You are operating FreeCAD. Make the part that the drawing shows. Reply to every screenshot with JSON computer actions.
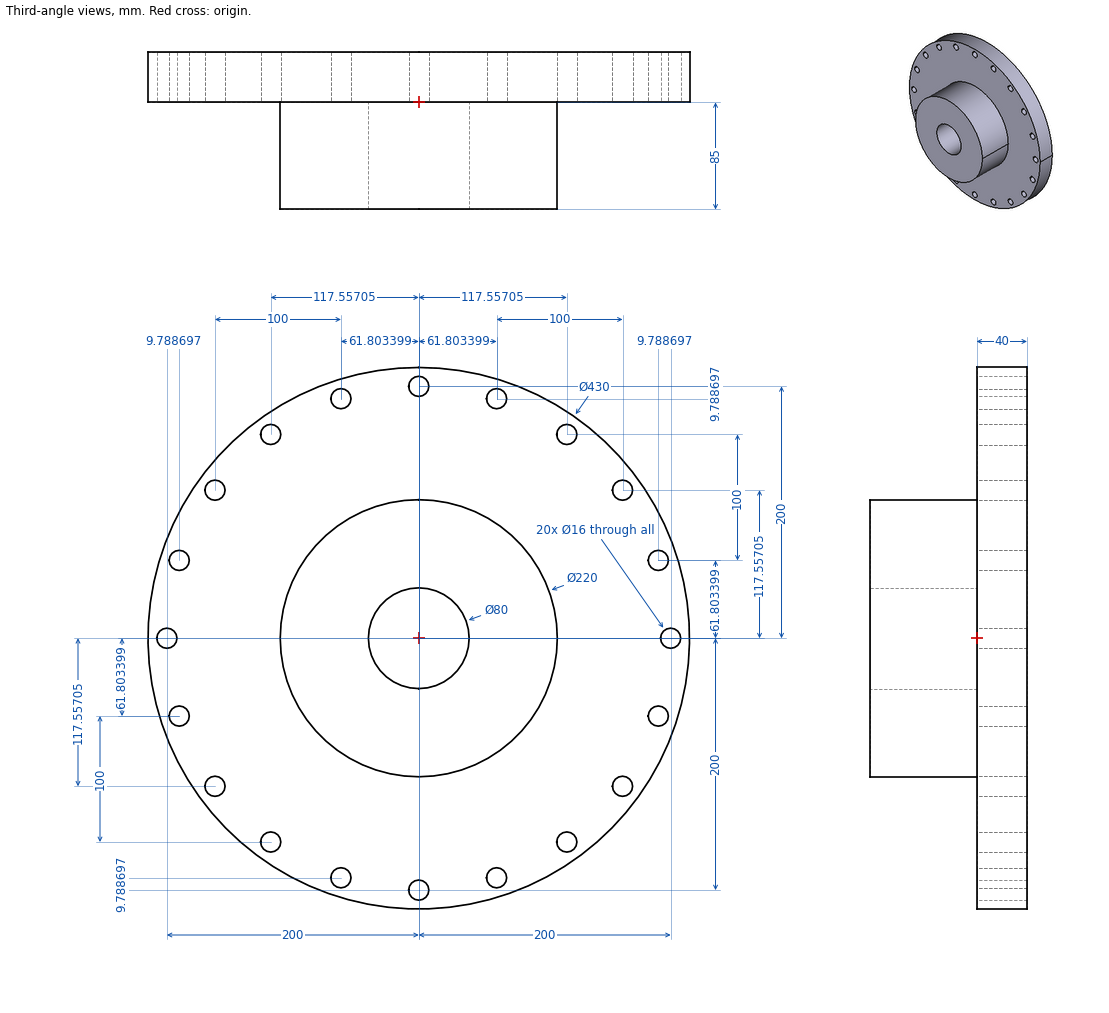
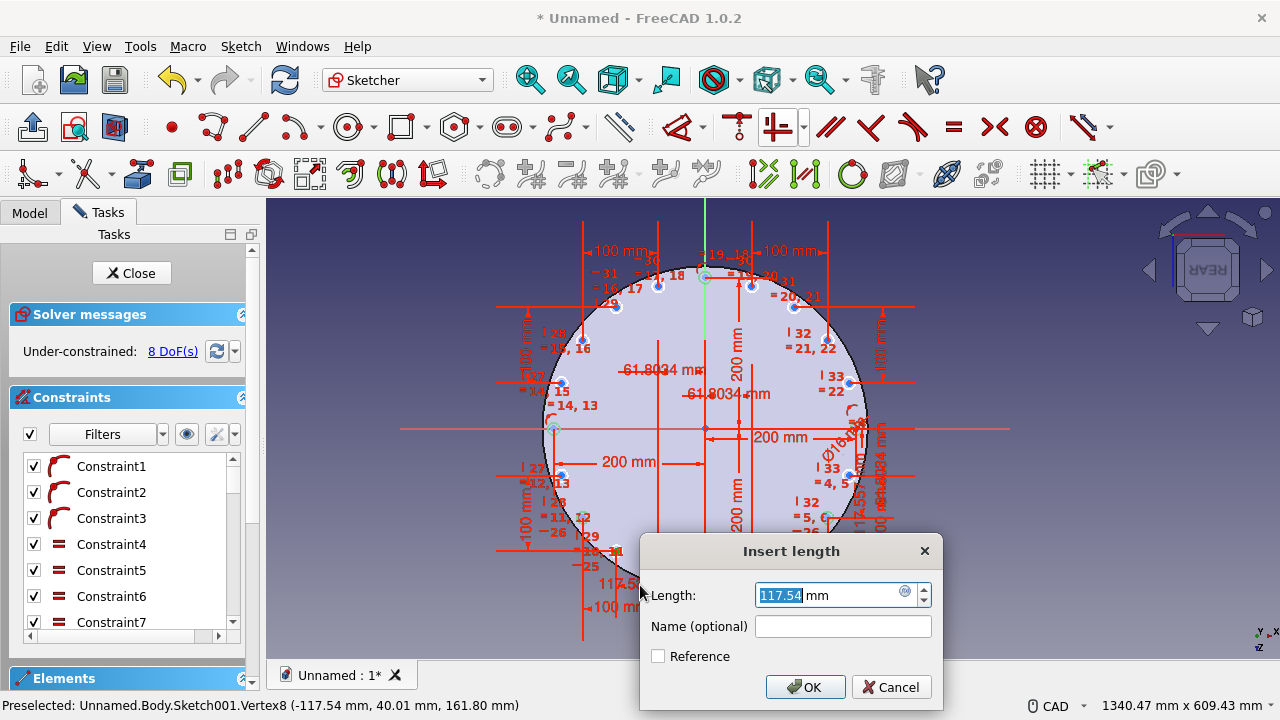
{"action": "type", "text": "117.55705"}
{"action": "key", "text": "Return"}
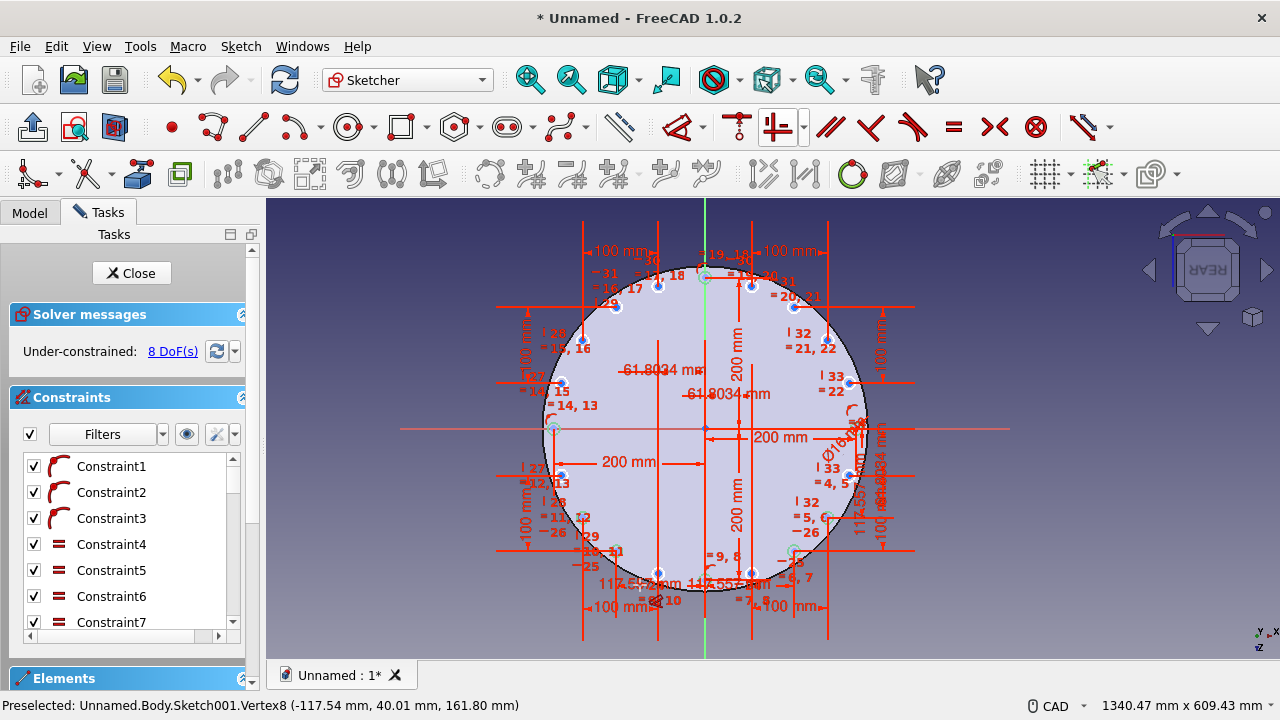
{"action": "left_click", "coordinate": [562, 383]}
{"action": "left_click", "coordinate": [528, 406]}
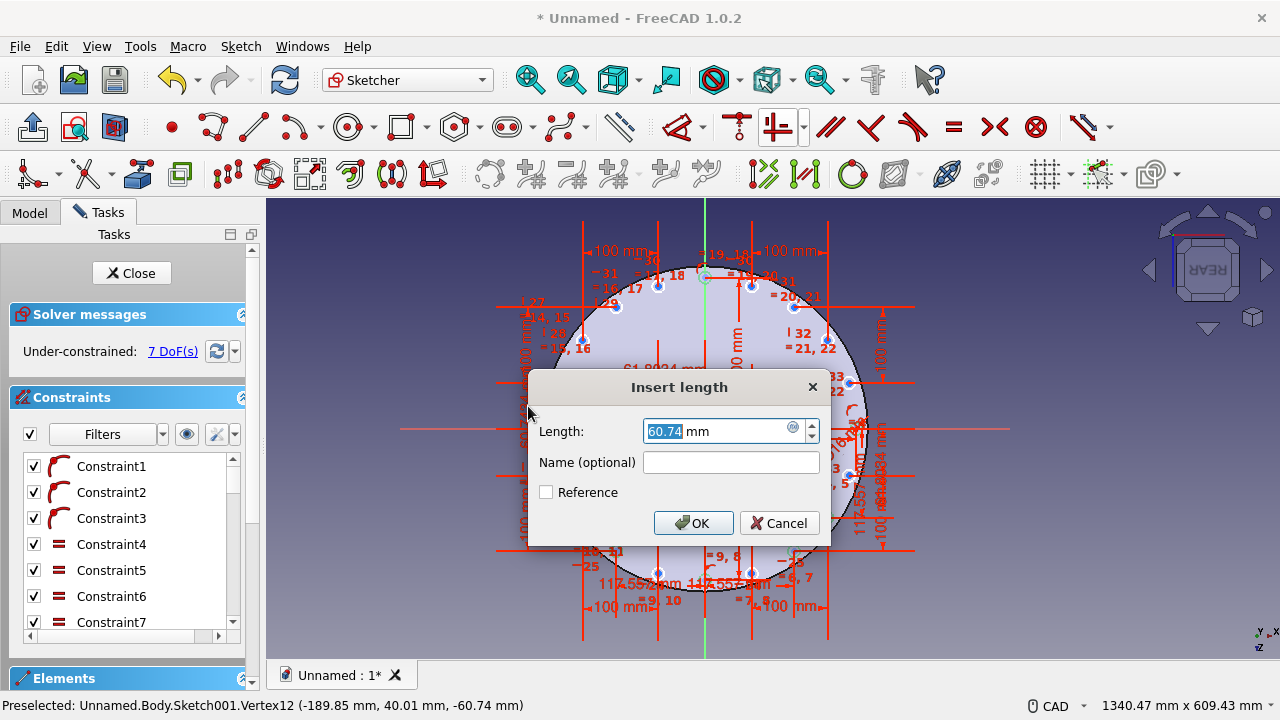
{"action": "type", "text": "61.803399"}
{"action": "key", "text": "Return"}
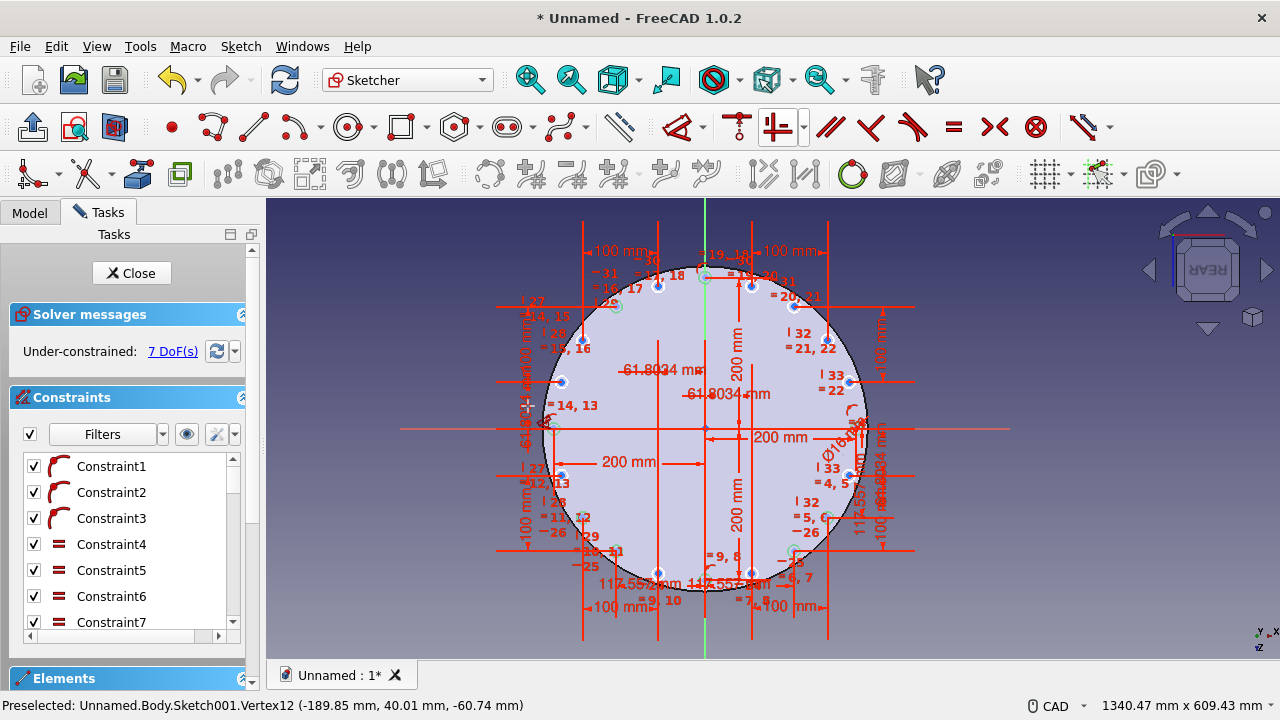
{"action": "left_click", "coordinate": [583, 341]}
{"action": "left_click", "coordinate": [739, 416]}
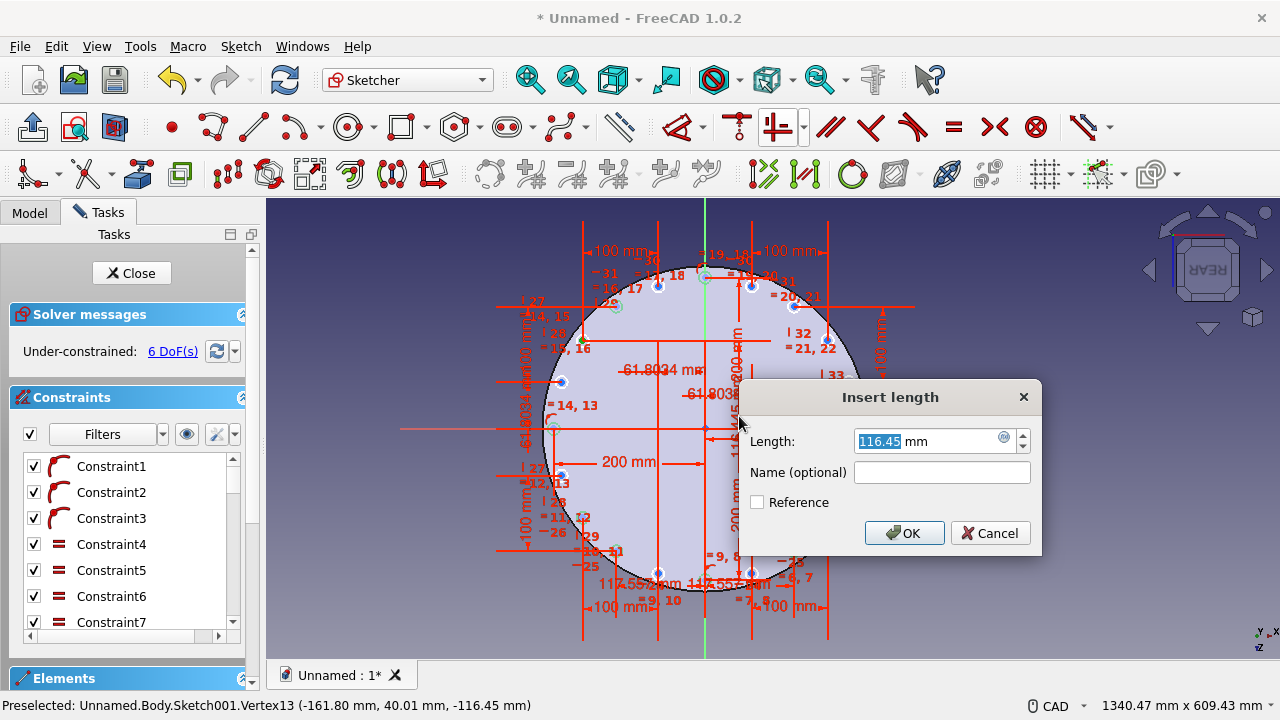
{"action": "type", "text": "117.55705"}
{"action": "key", "text": "Return"}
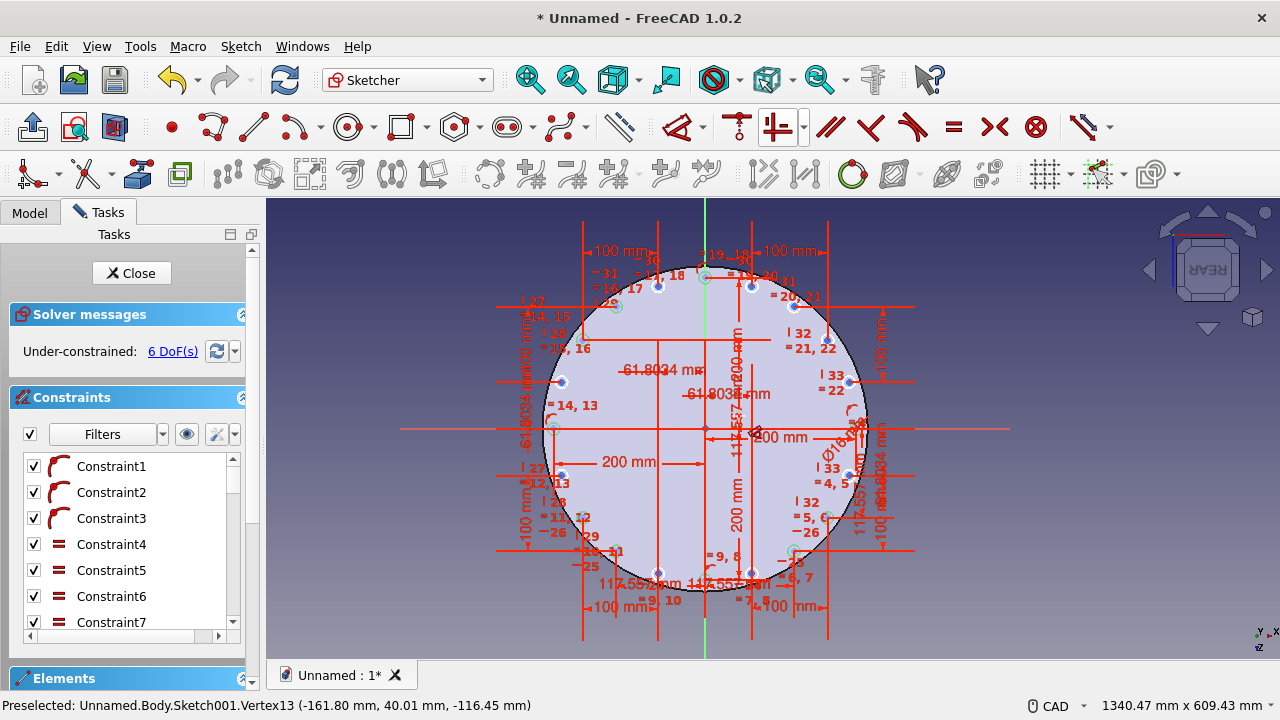
{"action": "left_click", "coordinate": [794, 307]}
{"action": "left_click", "coordinate": [729, 273]}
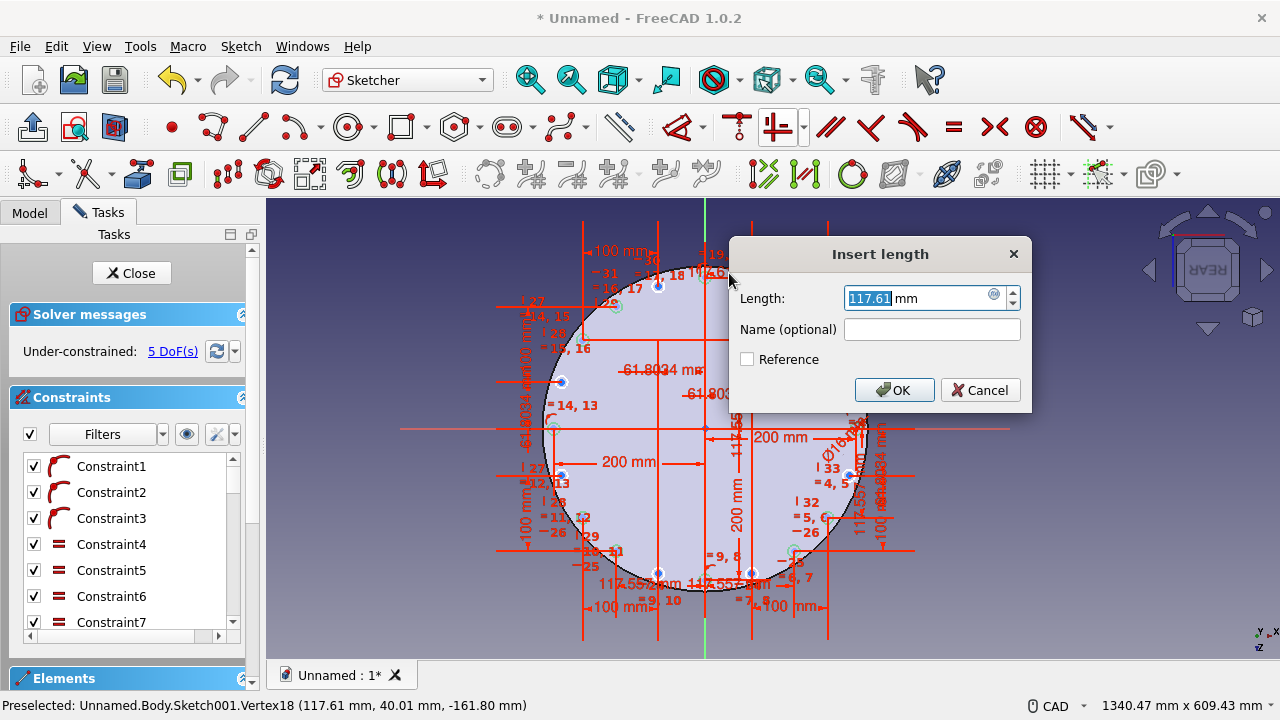
{"action": "type", "text": "117.55705"}
{"action": "key", "text": "Return"}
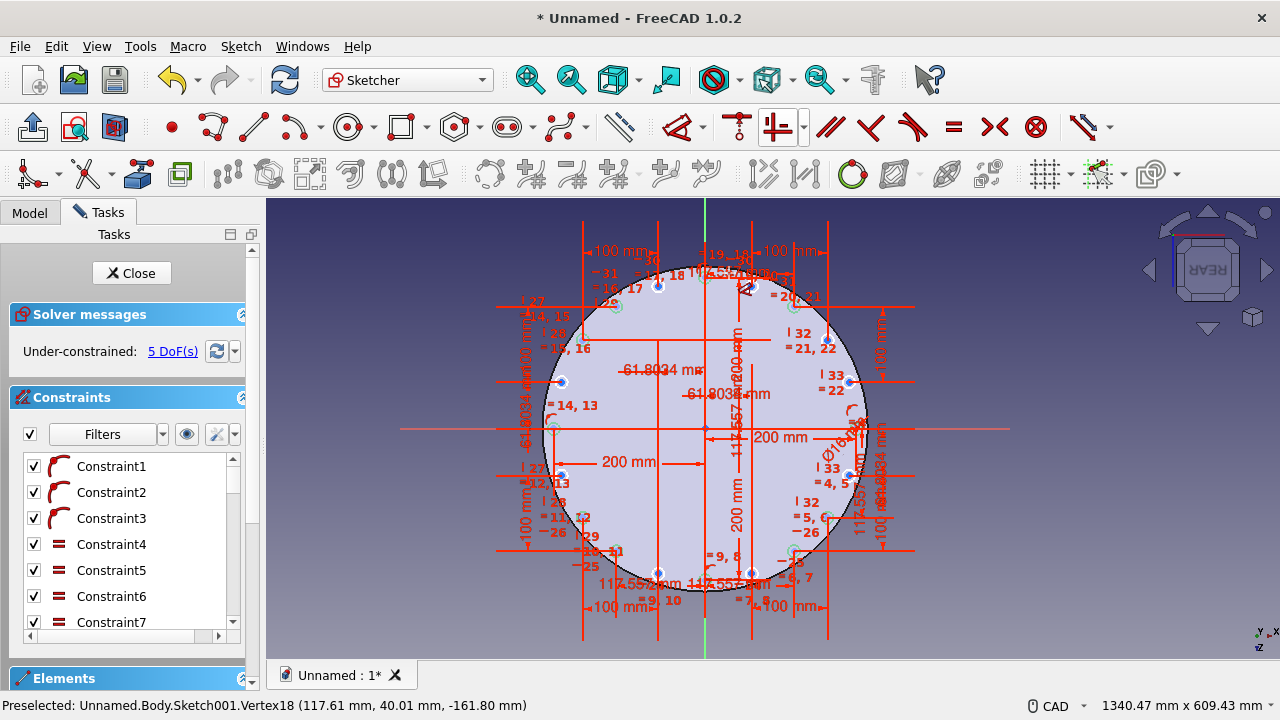
{"action": "left_click", "coordinate": [828, 340]}
{"action": "left_click", "coordinate": [862, 405]}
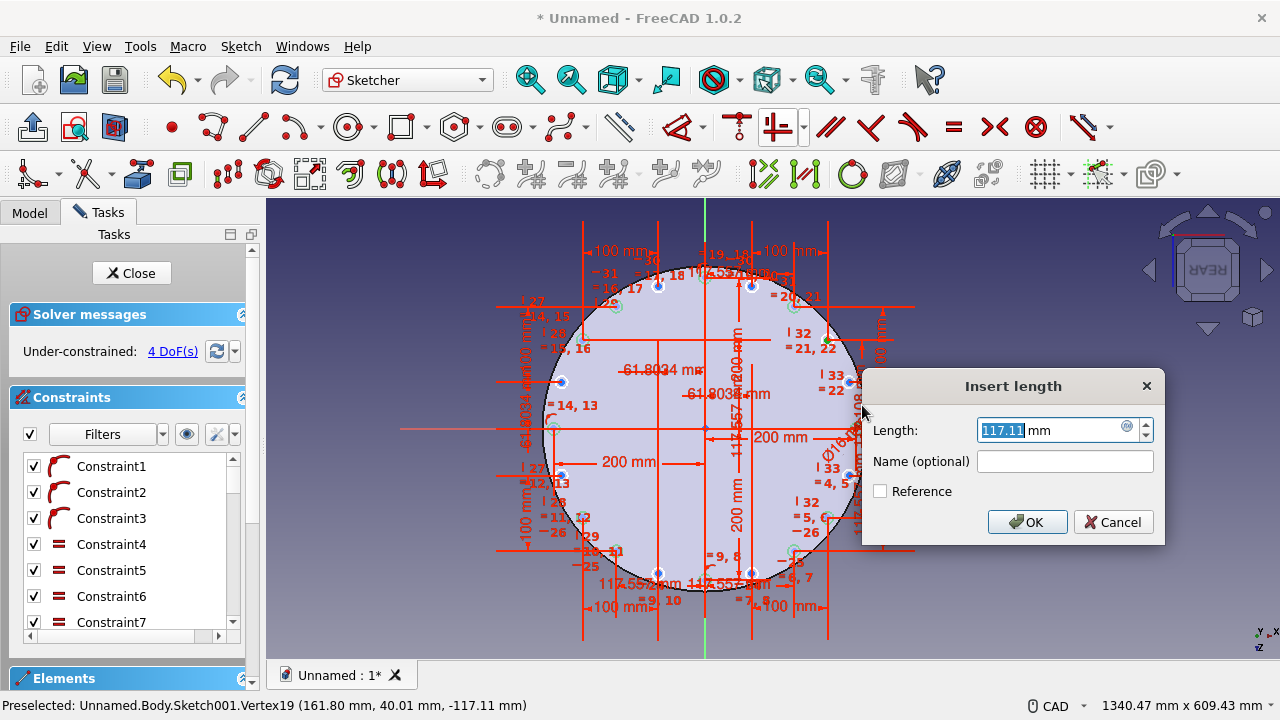
{"action": "type", "text": "117.55705"}
{"action": "key", "text": "Return"}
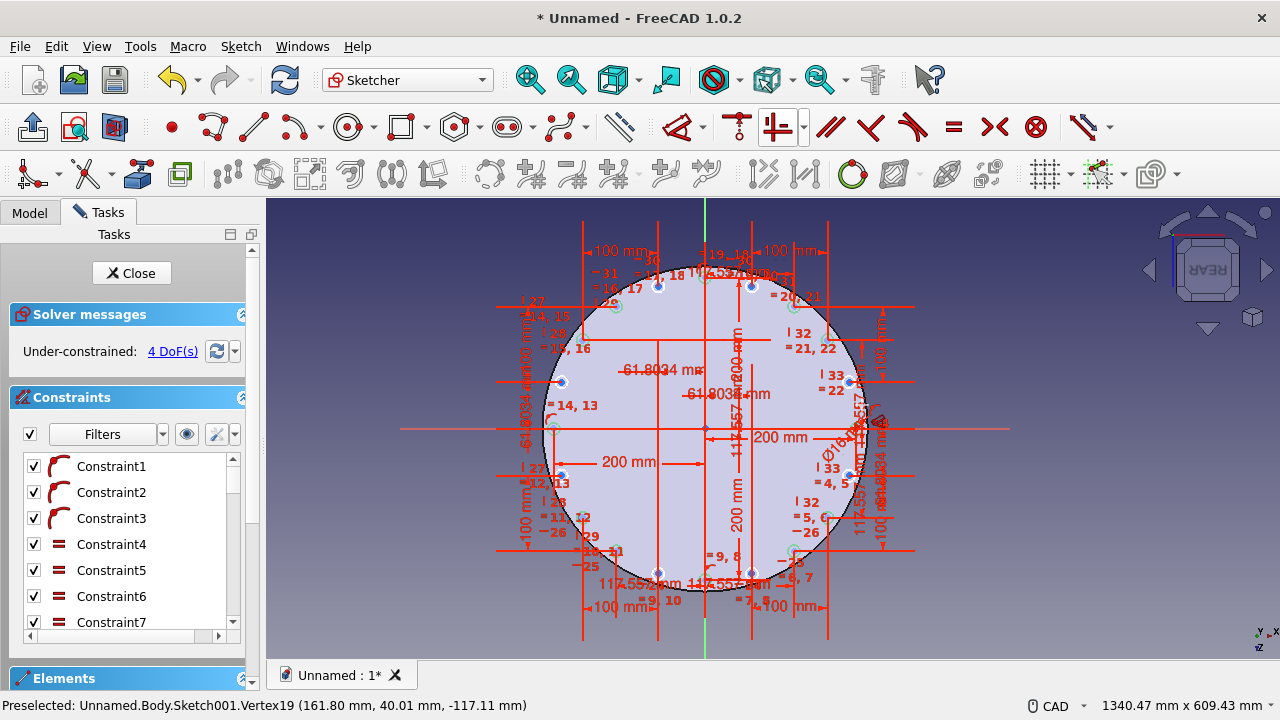
{"action": "scroll", "coordinate": [856, 429], "scroll_direction": "up", "scroll_amount": 9}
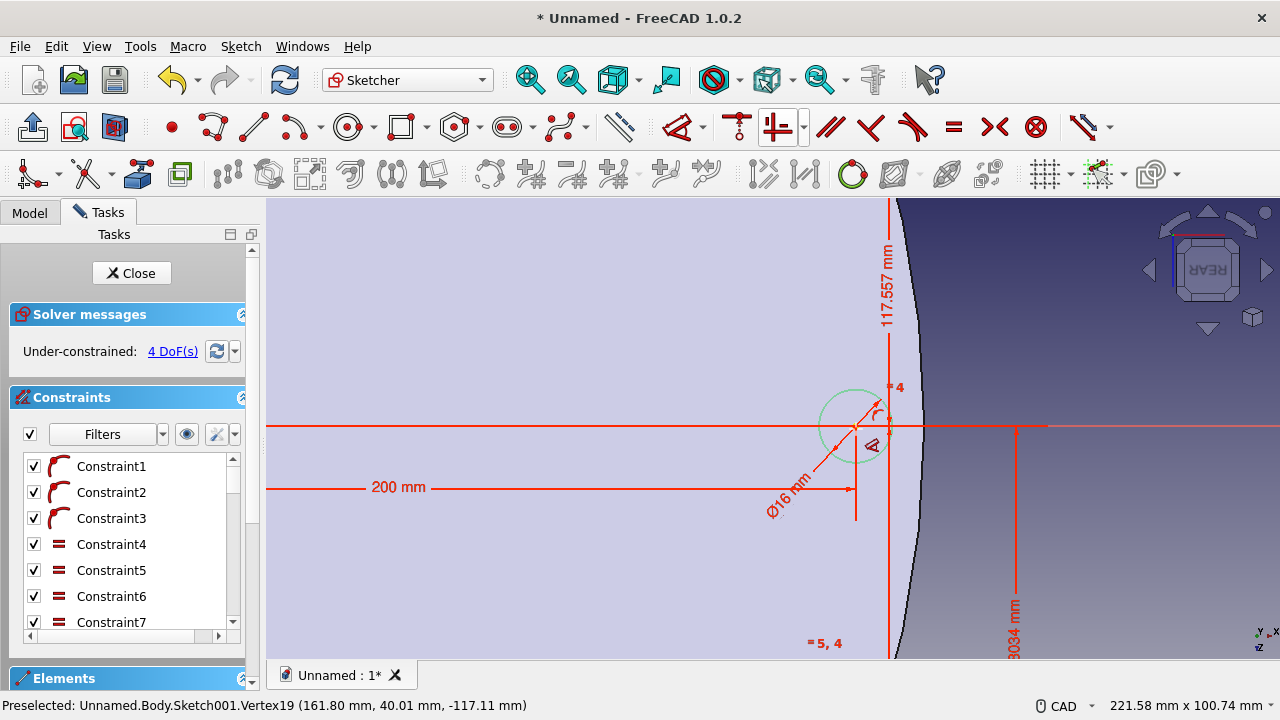
{"action": "left_click", "coordinate": [856, 426]}